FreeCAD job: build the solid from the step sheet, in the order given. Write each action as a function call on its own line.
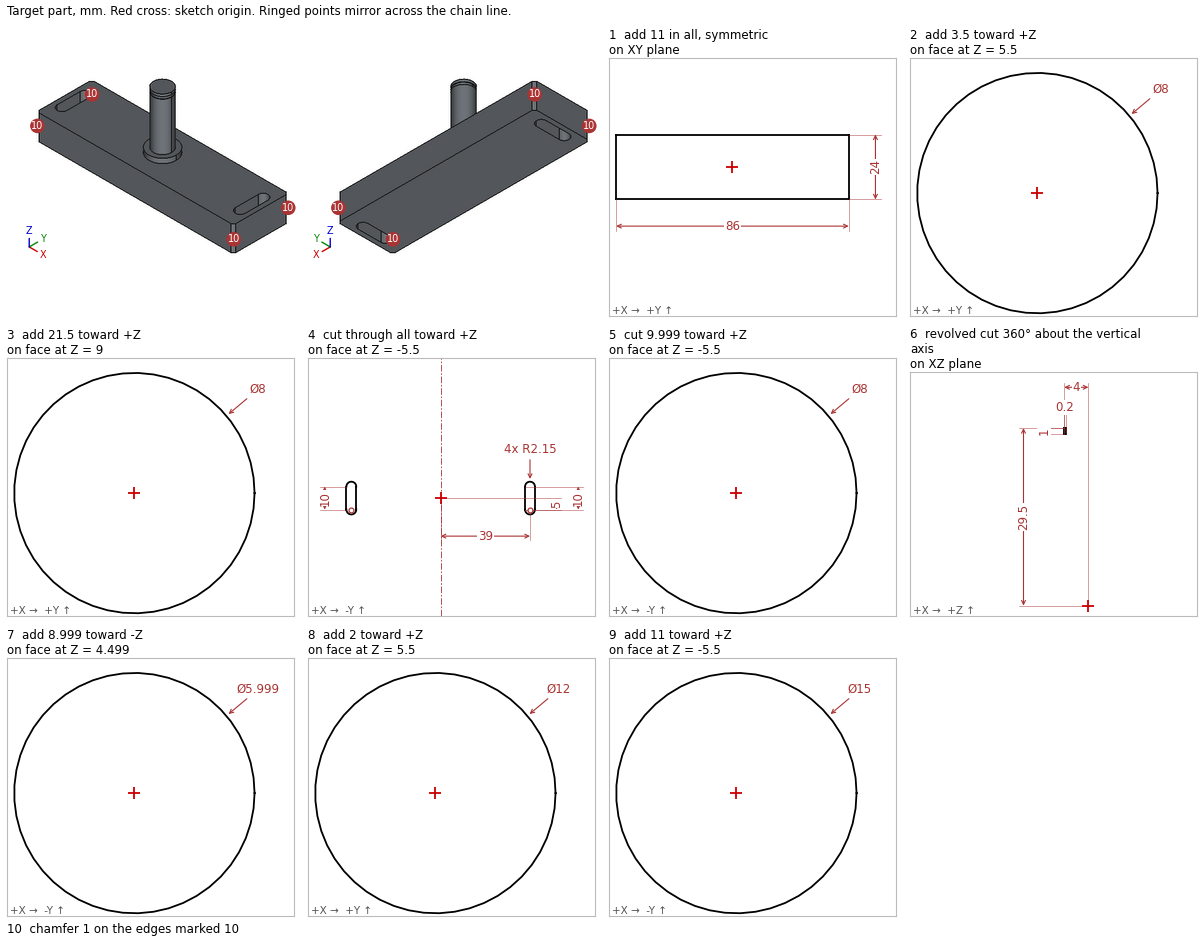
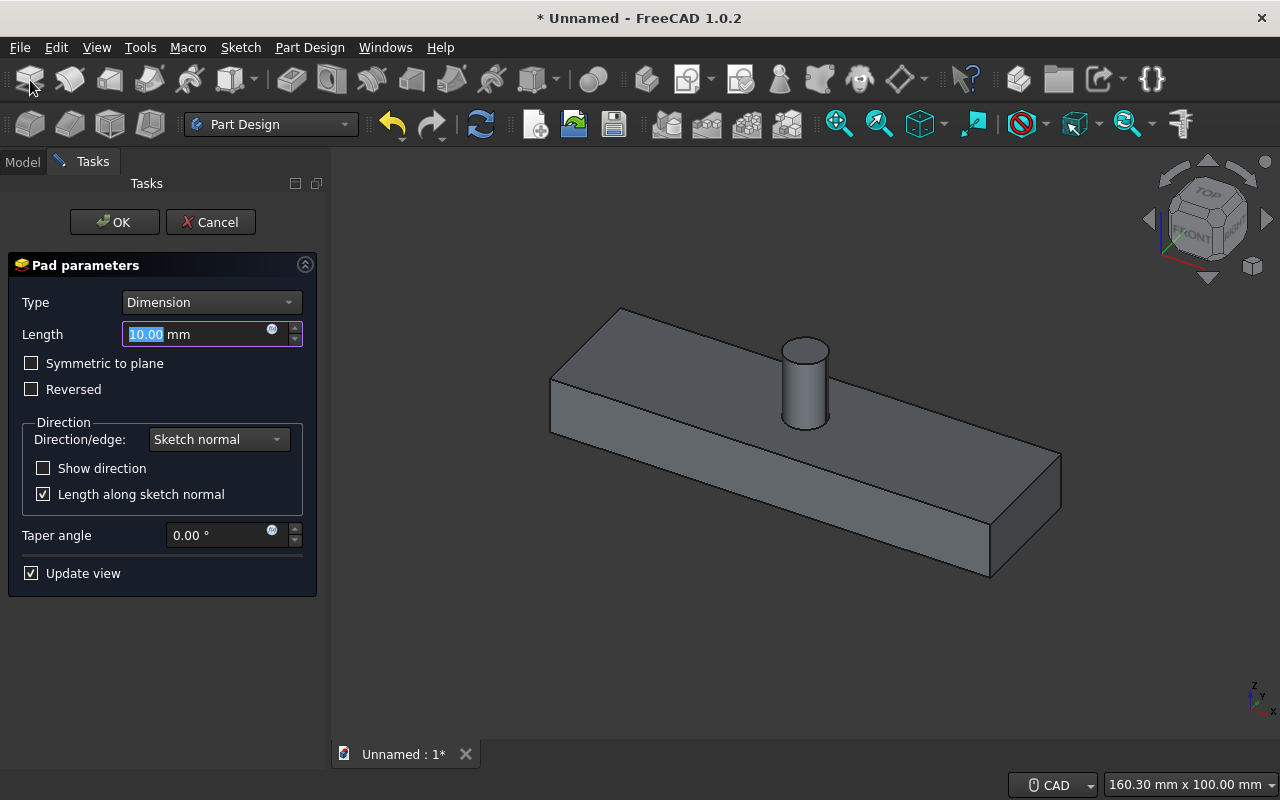
text(21.5)
key(Tab)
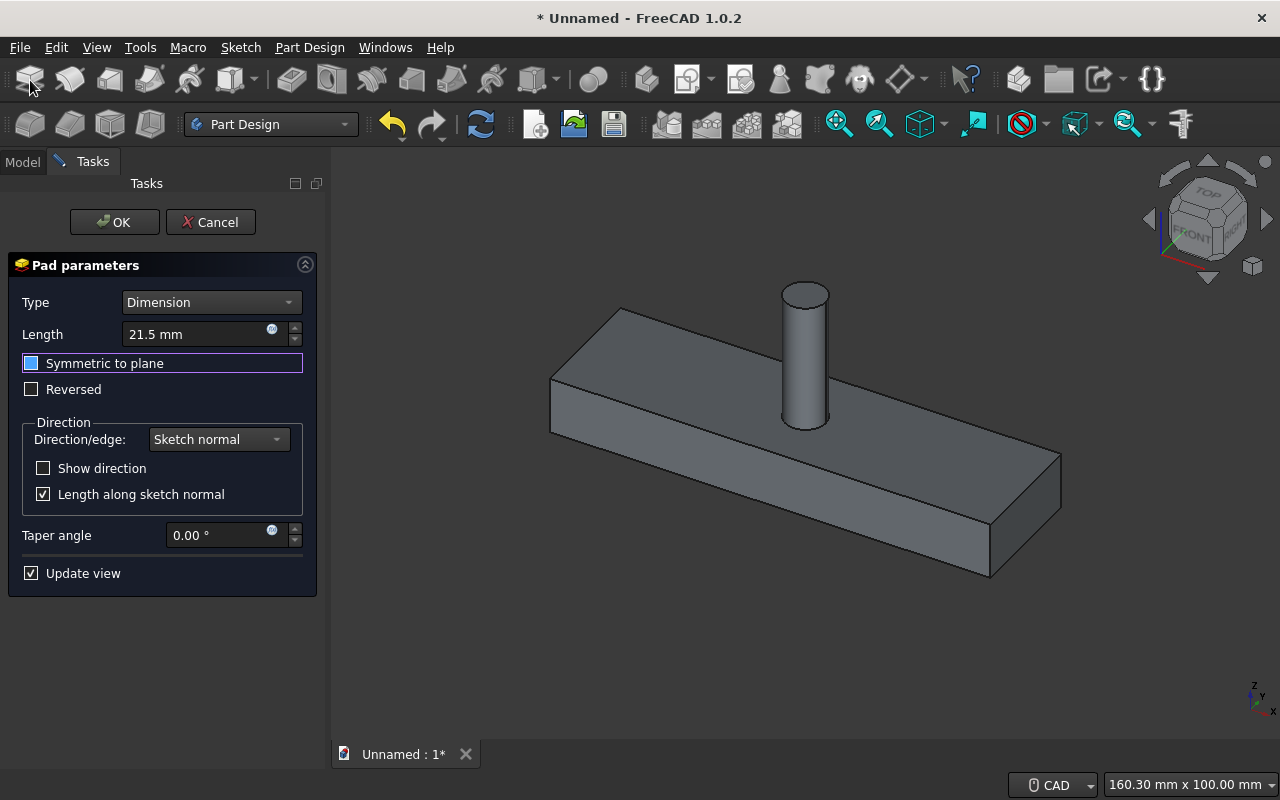
click(115, 222)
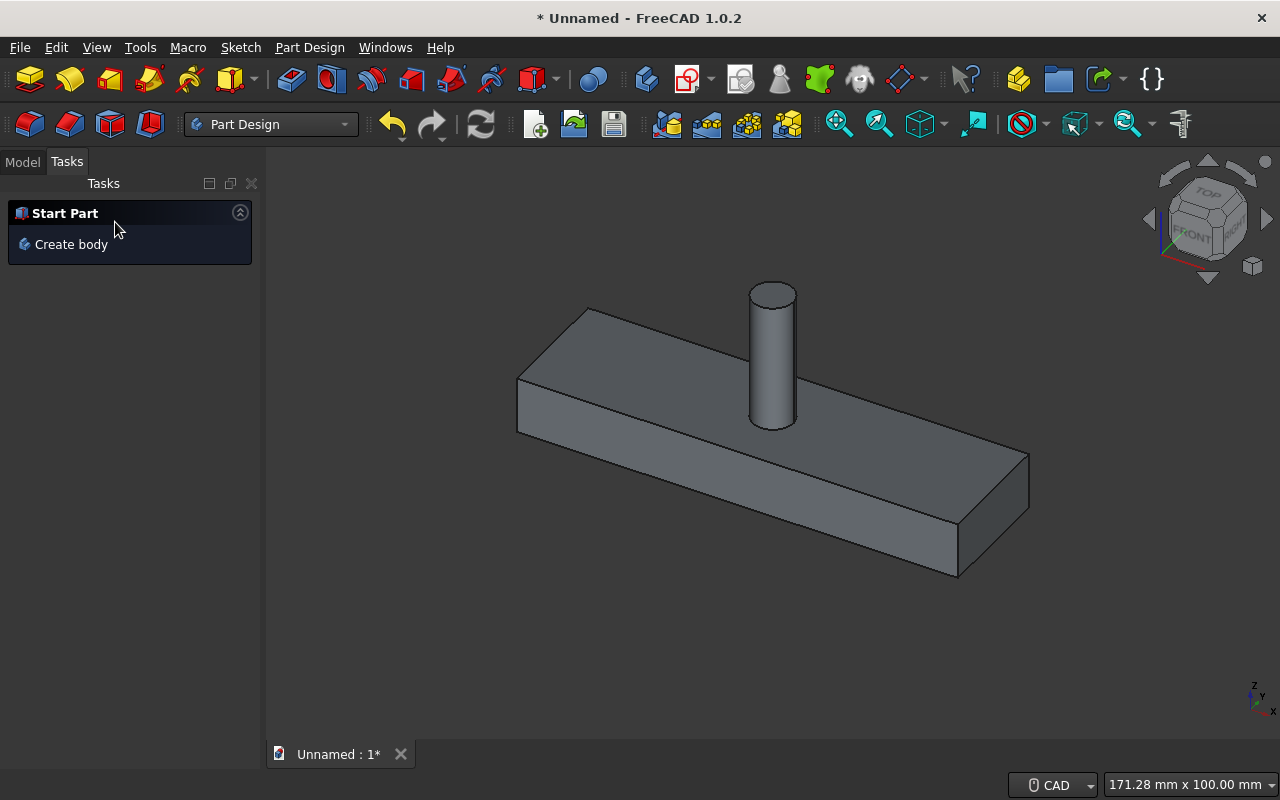
key(5)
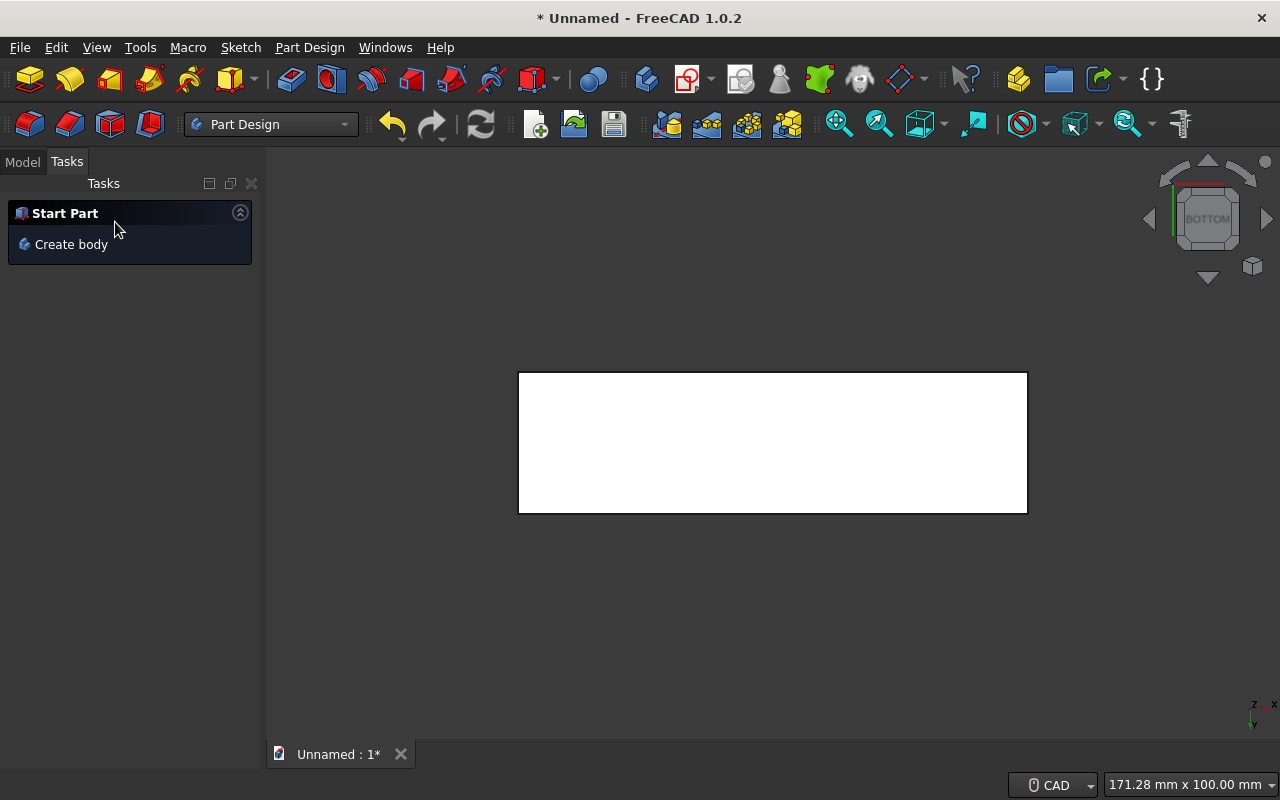
click(918, 442)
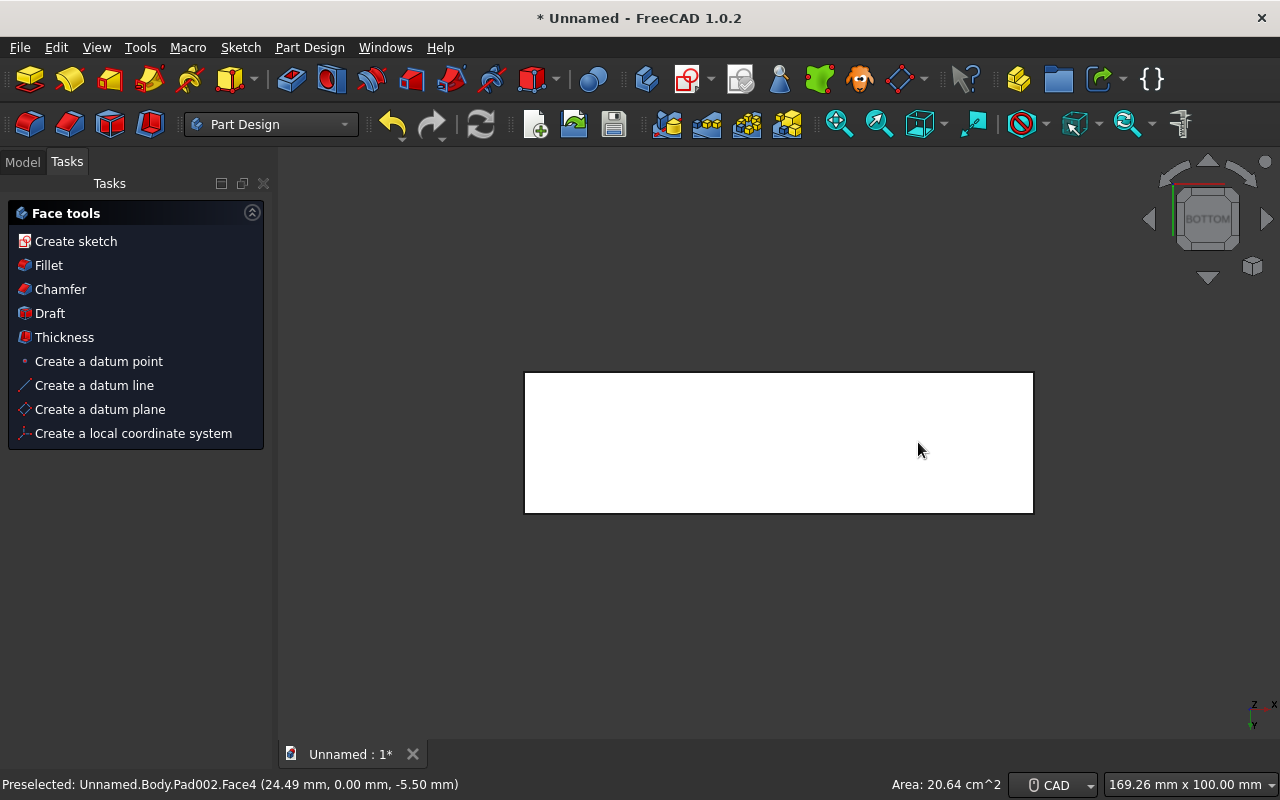
click(688, 80)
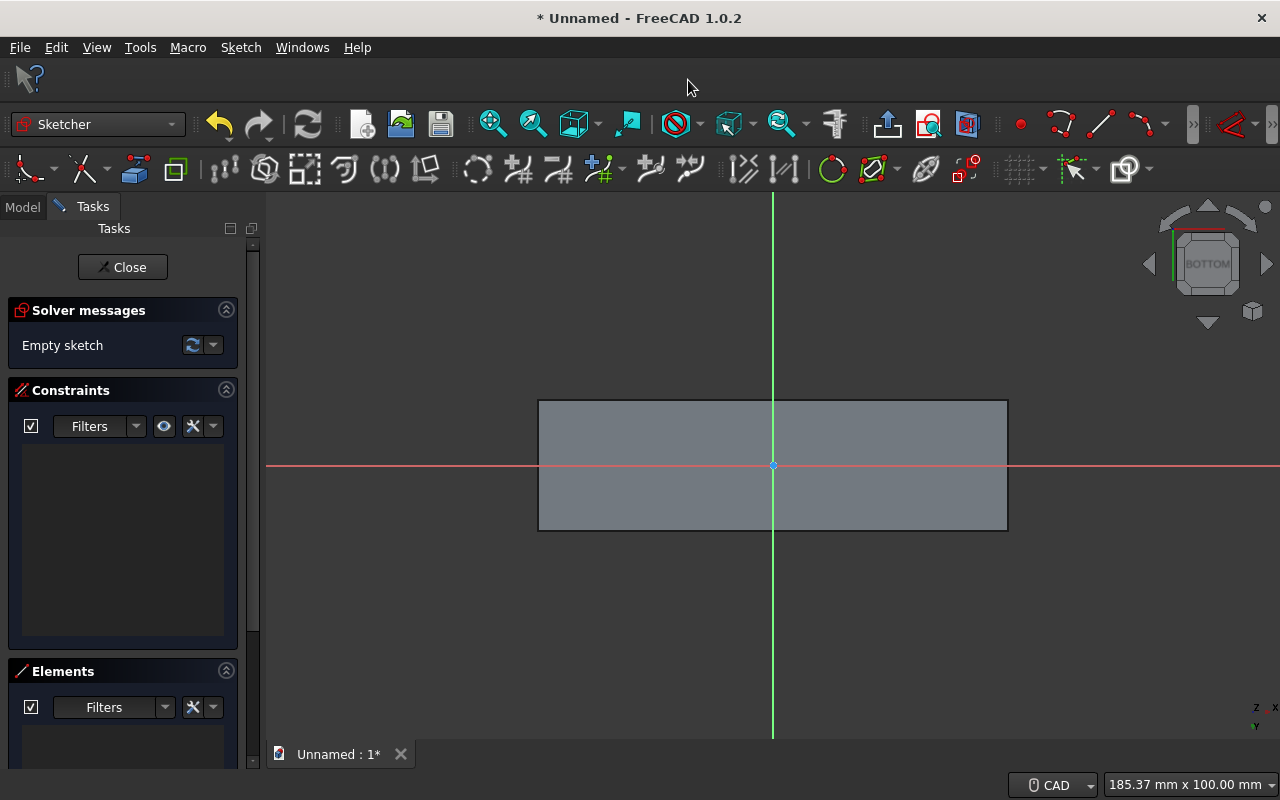
key(g)
key(s)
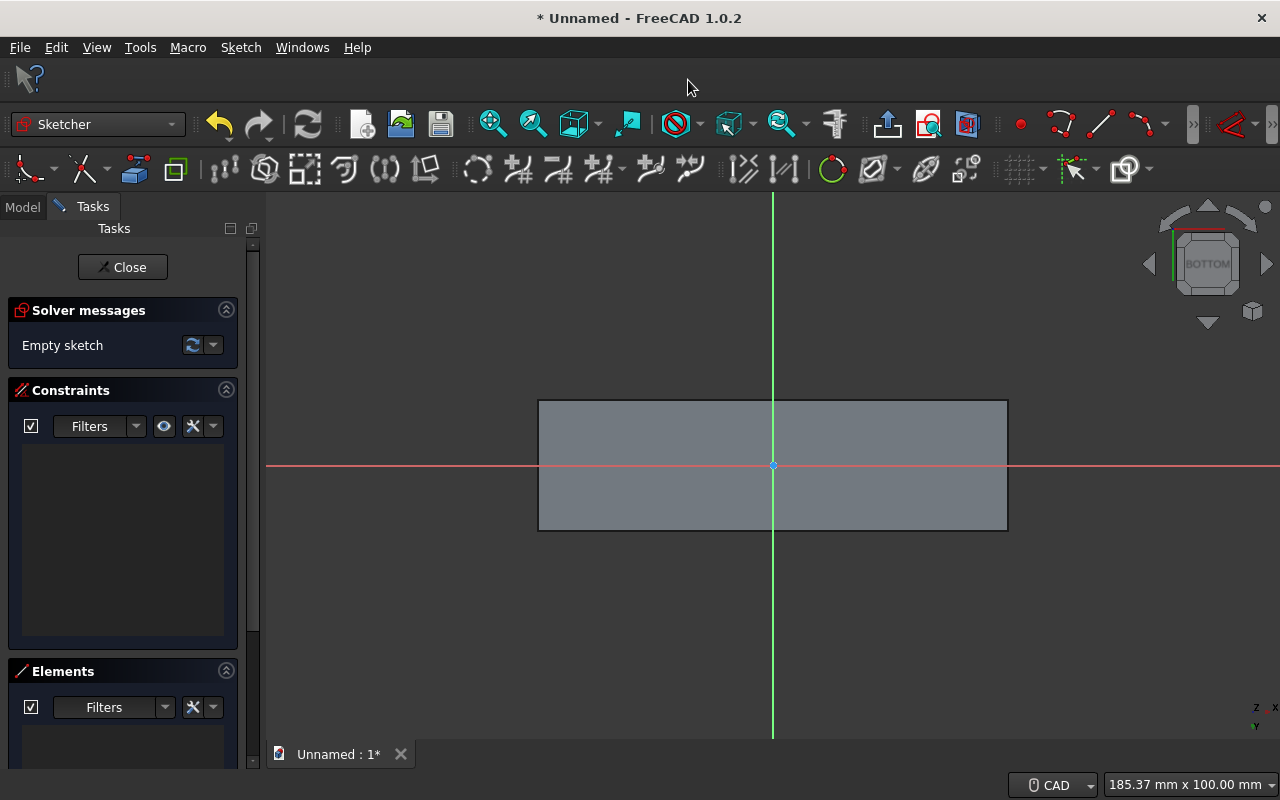
scroll(986, 493, up, 4)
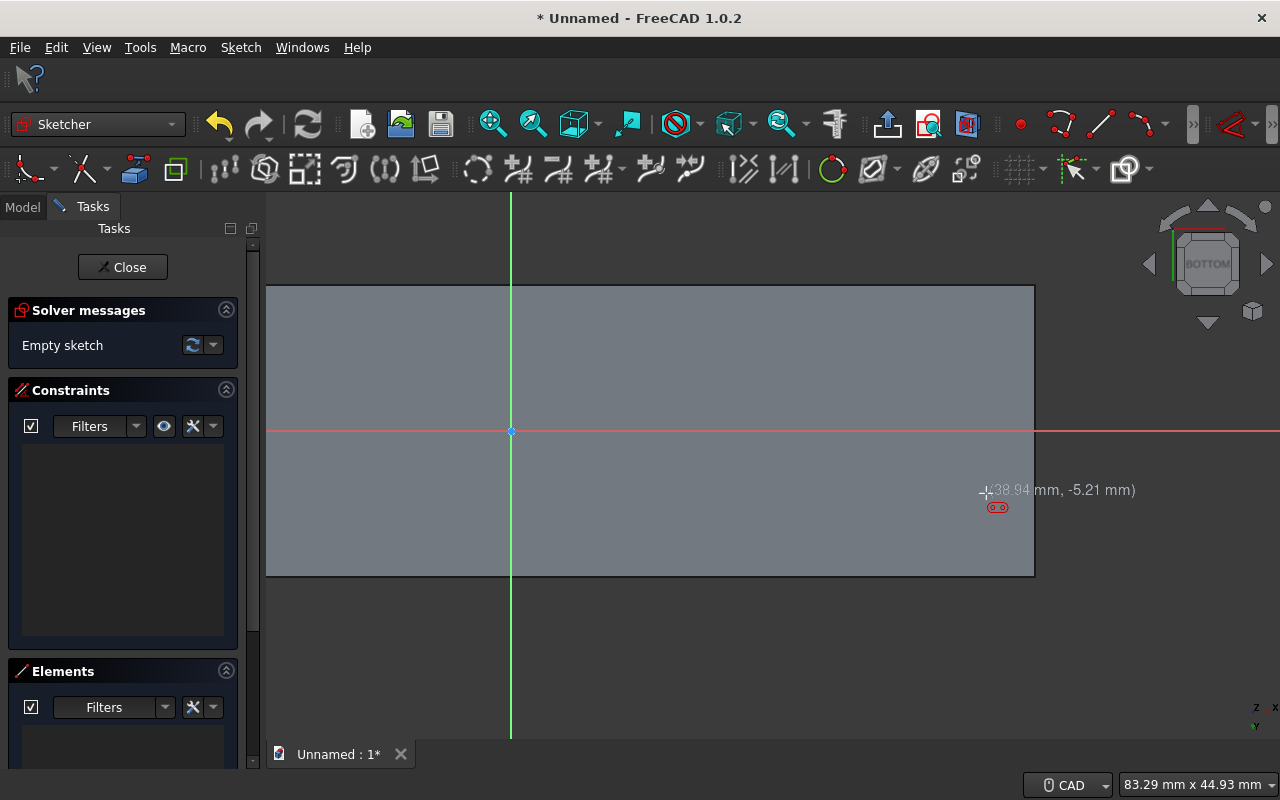
click(986, 492)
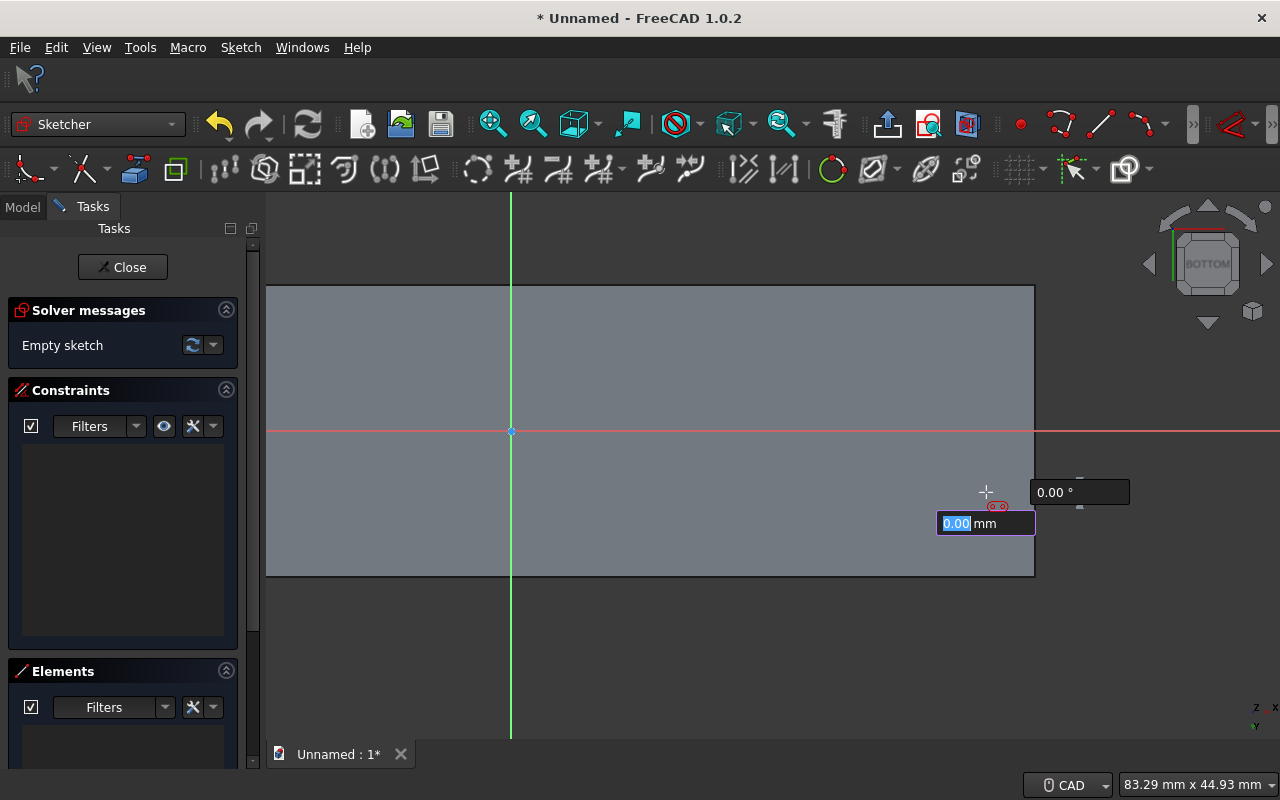
click(986, 370)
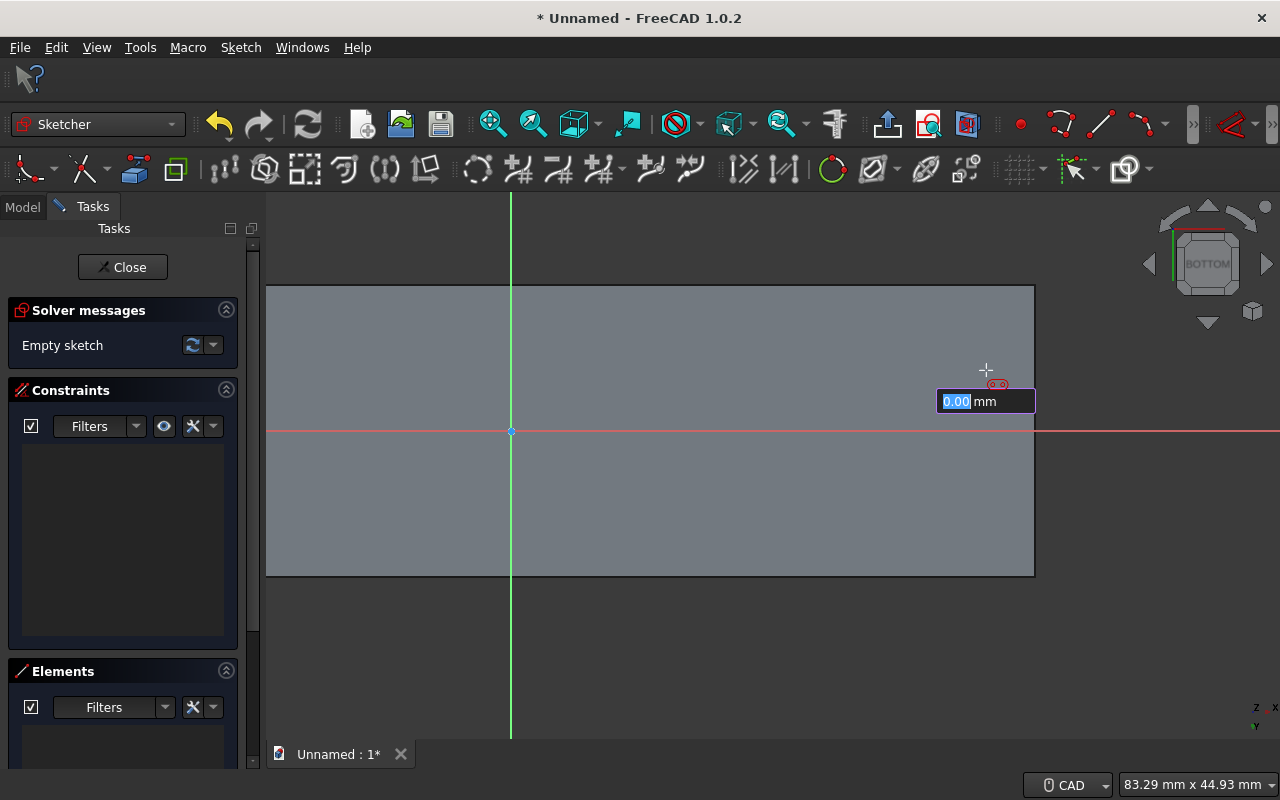
click(960, 413)